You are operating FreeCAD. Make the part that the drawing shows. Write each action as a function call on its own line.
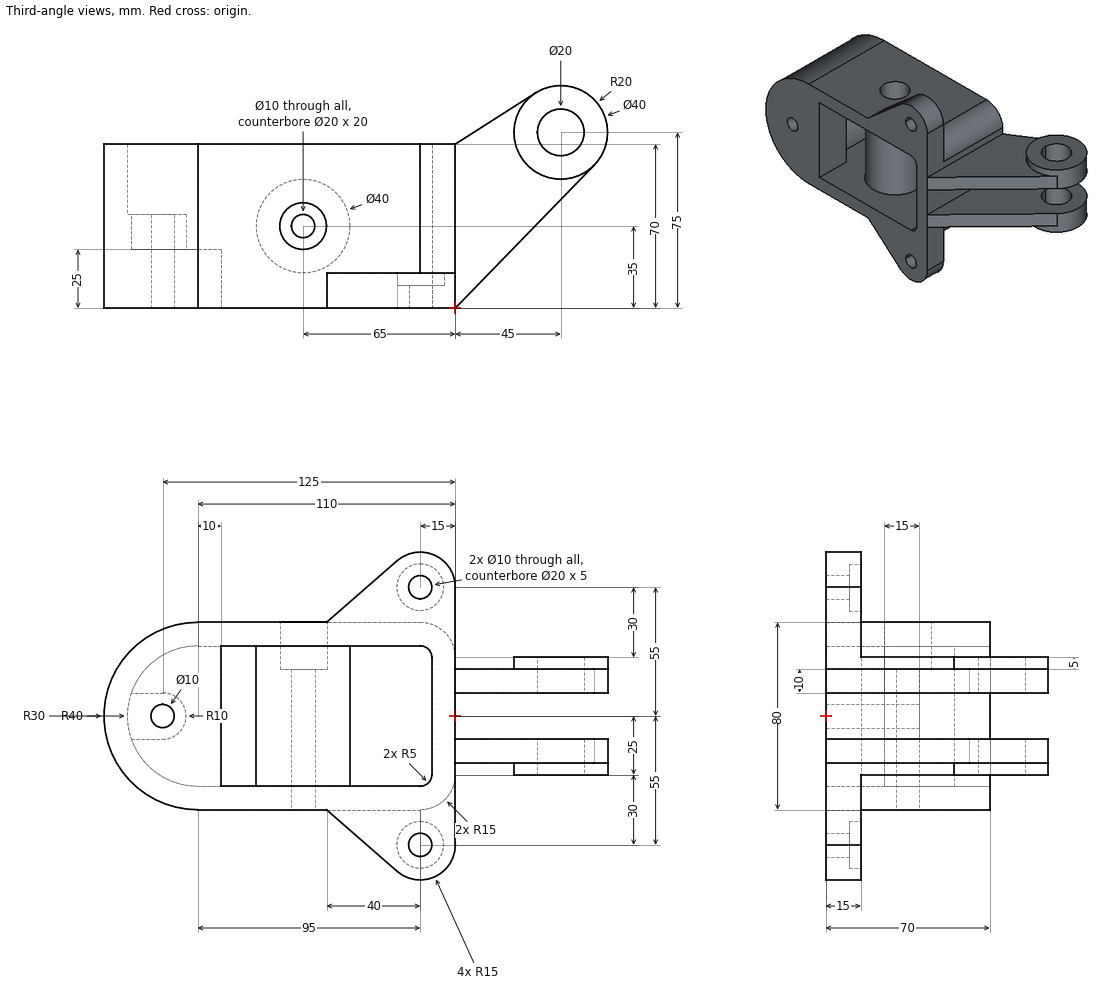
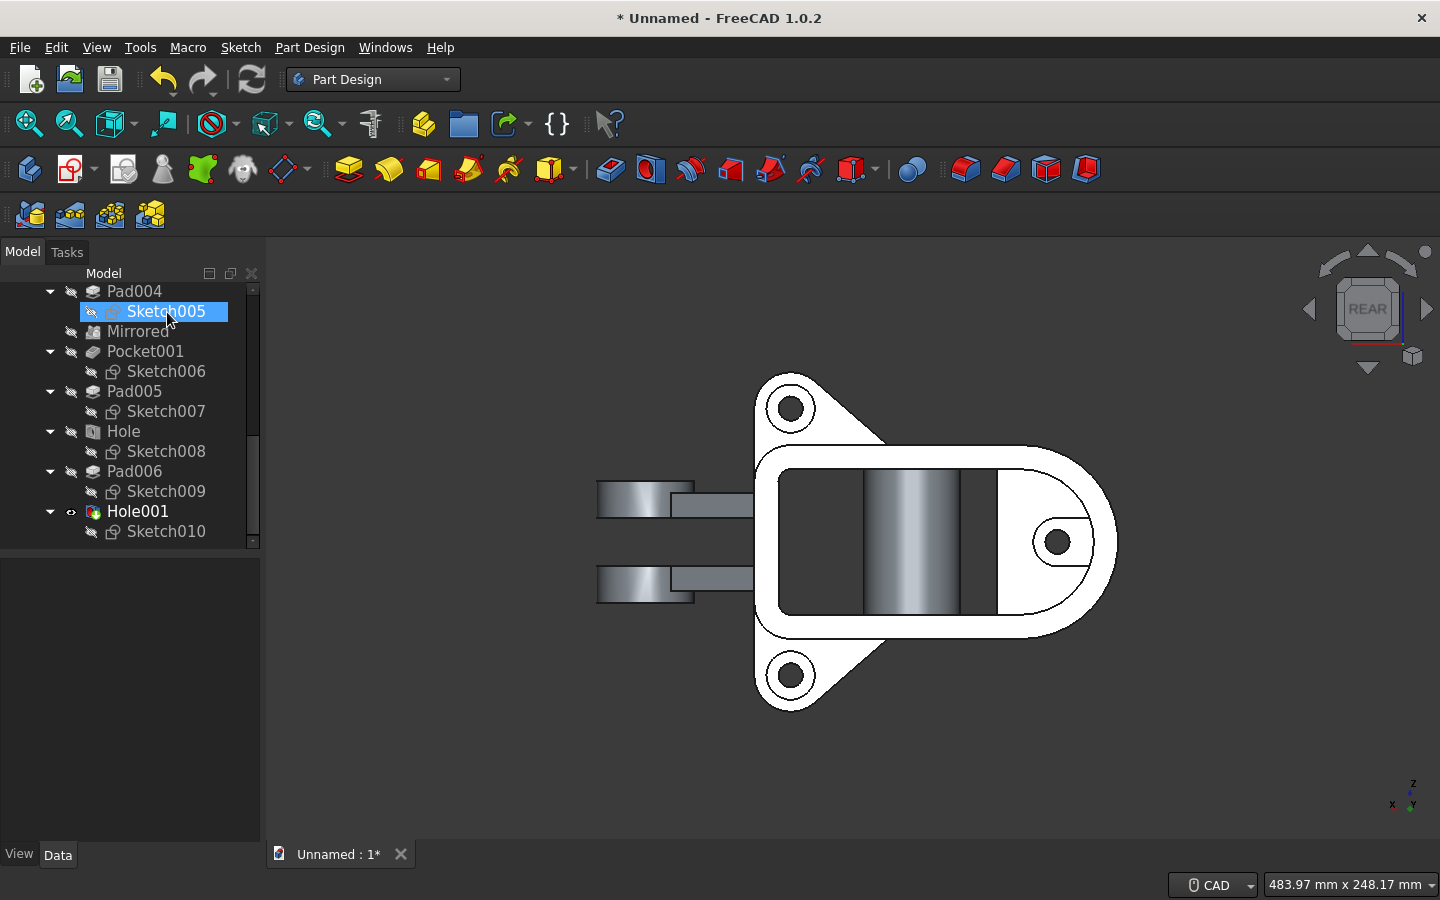
key(0)